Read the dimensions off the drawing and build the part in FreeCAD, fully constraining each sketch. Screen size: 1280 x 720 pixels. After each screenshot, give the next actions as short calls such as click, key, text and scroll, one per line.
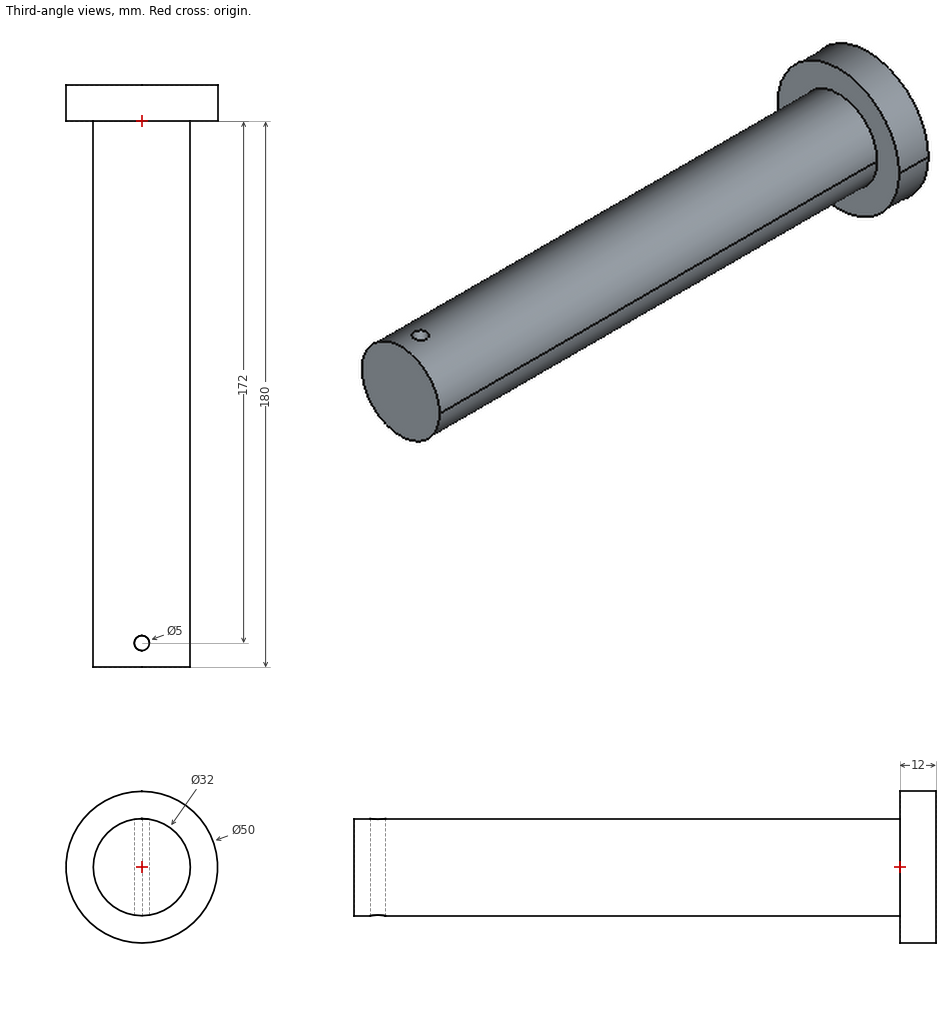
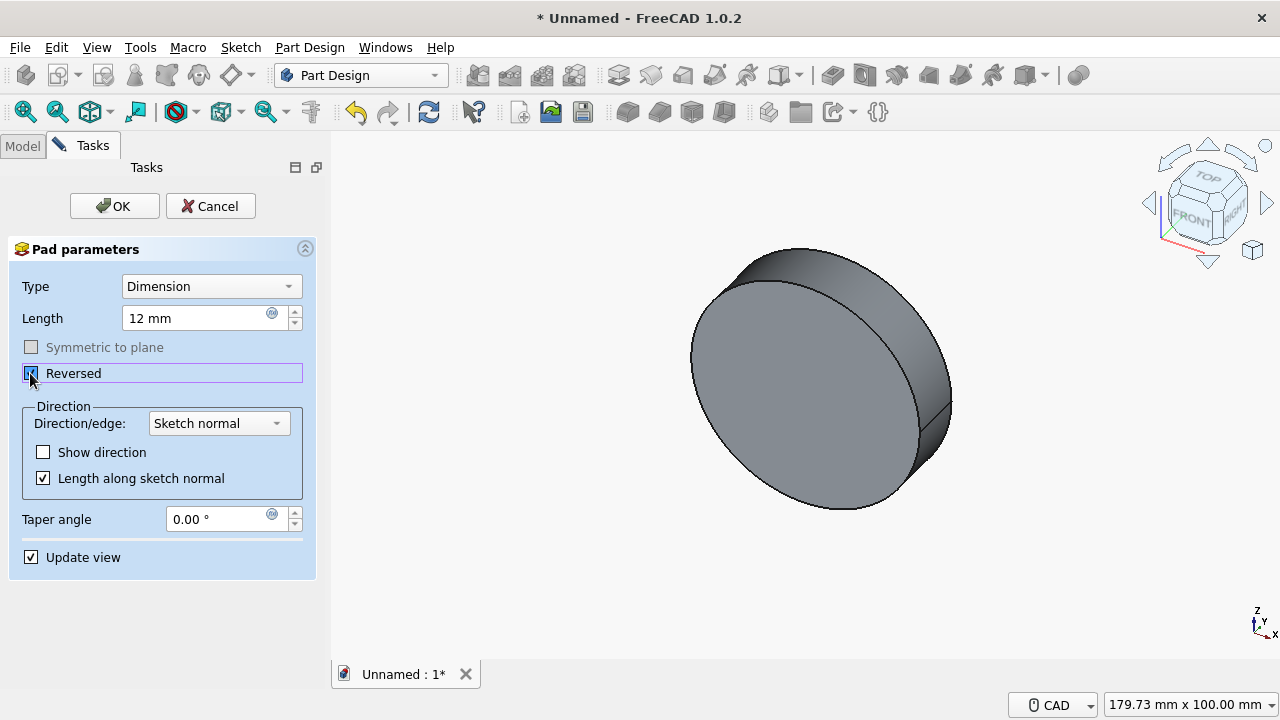
click(115, 206)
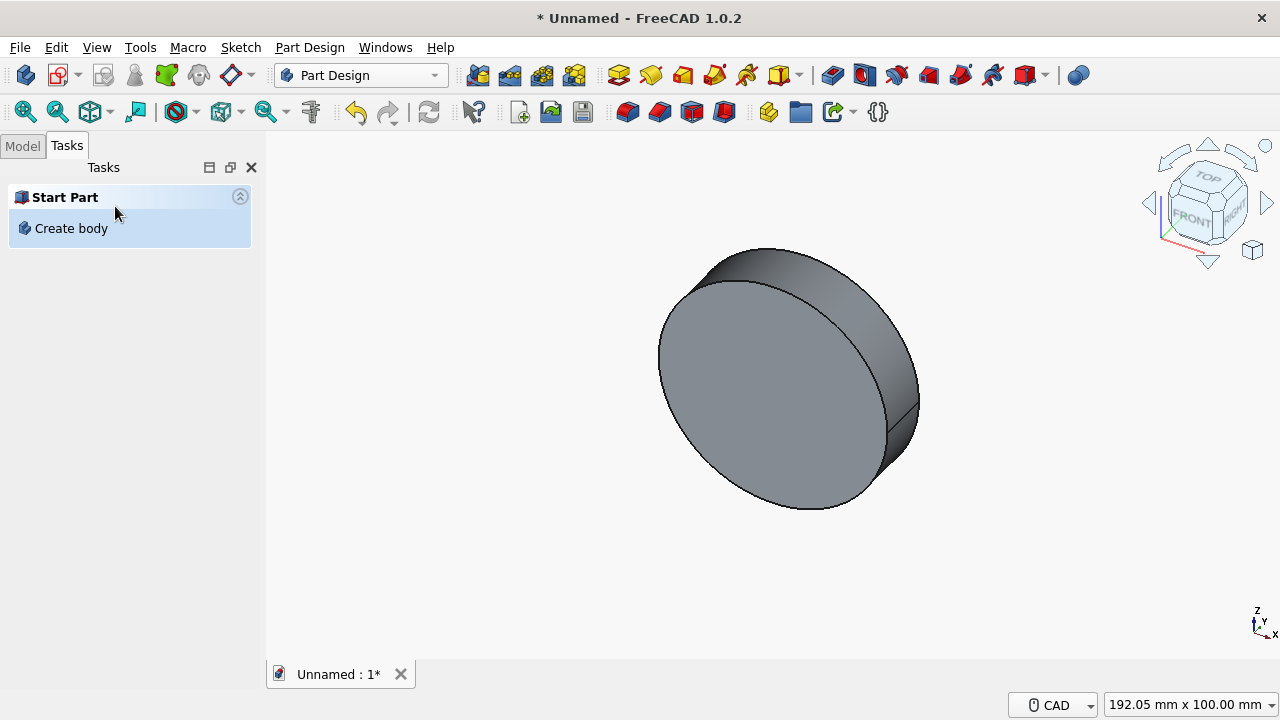
click(58, 76)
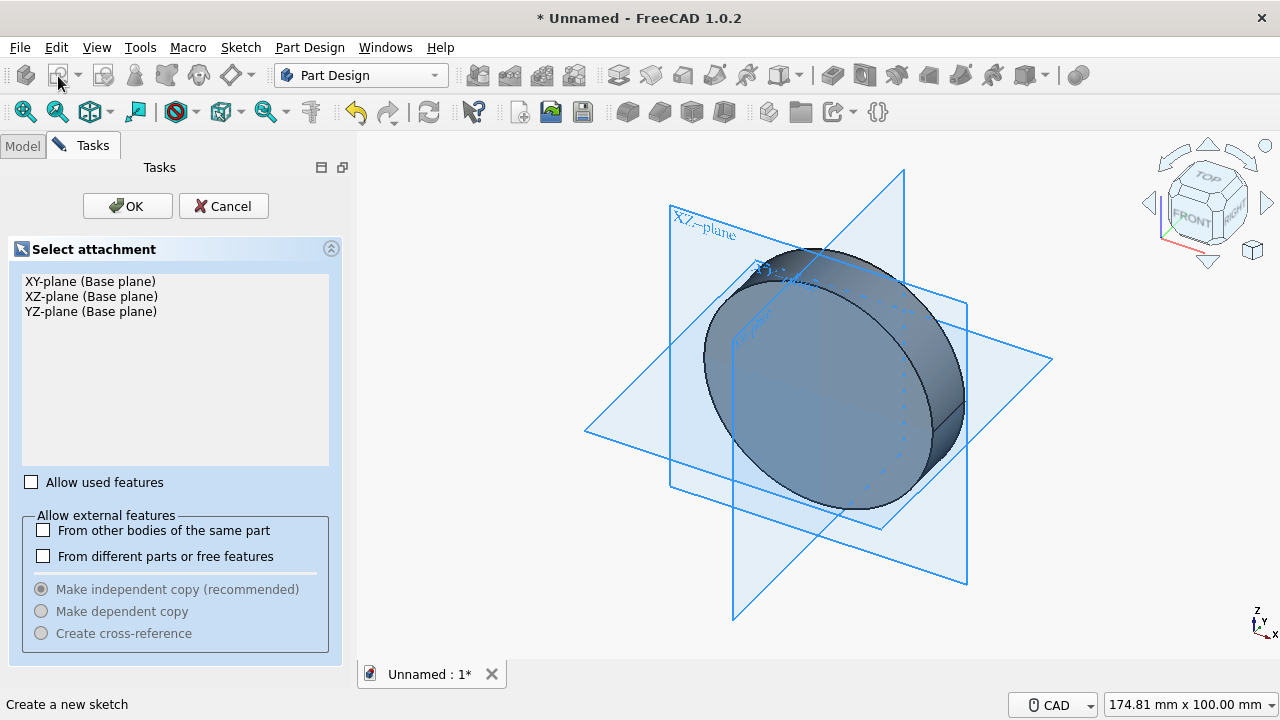
click(82, 296)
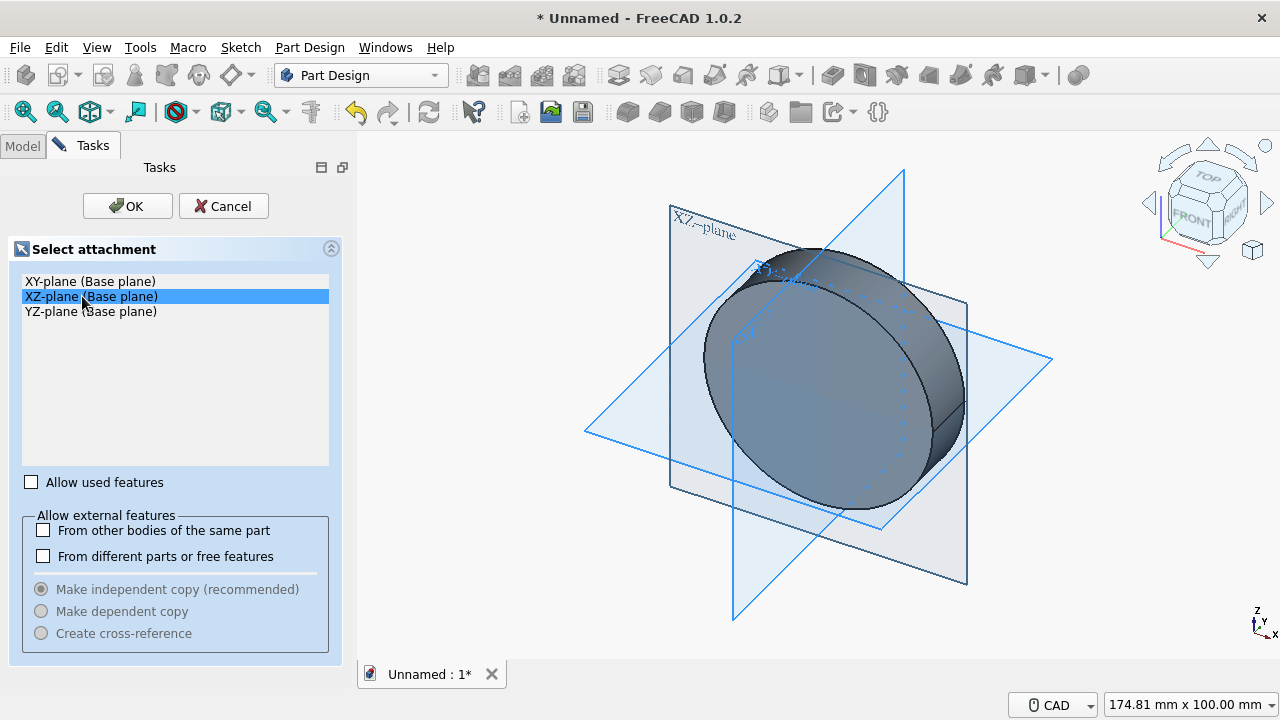
click(128, 206)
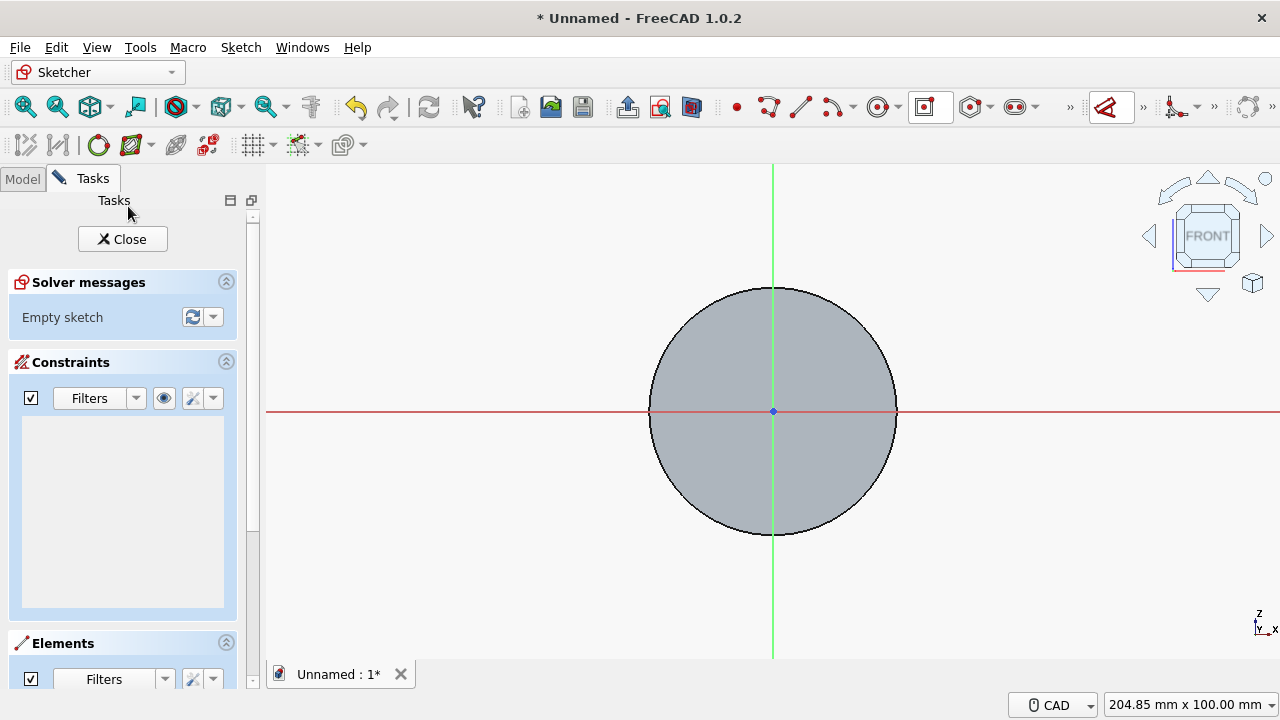
scroll(856, 412, up, 3)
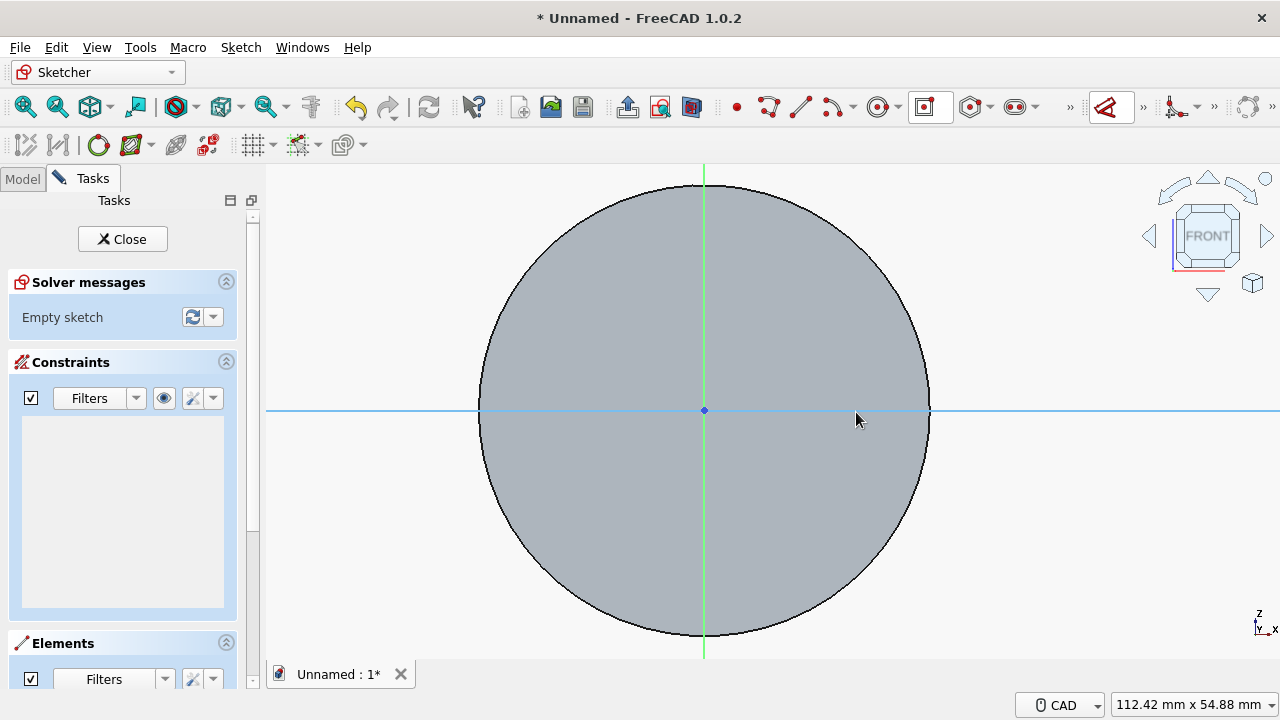
click(878, 108)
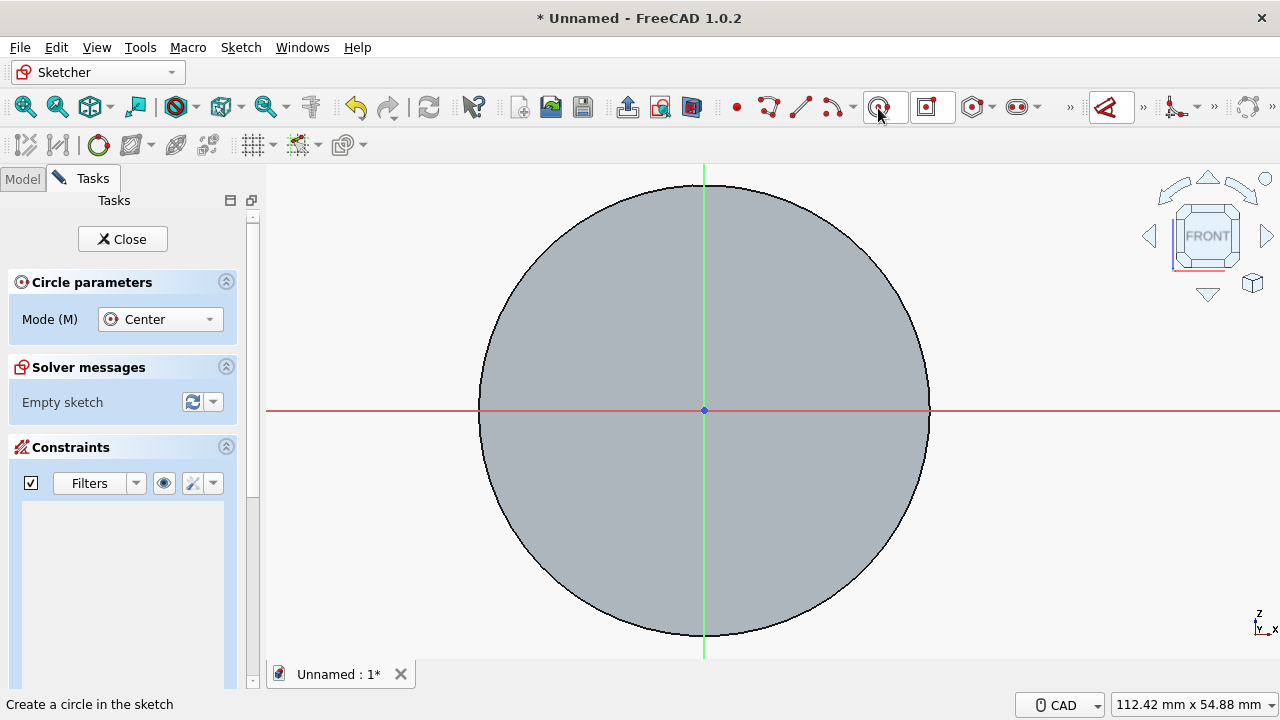
click(704, 411)
move(806, 309)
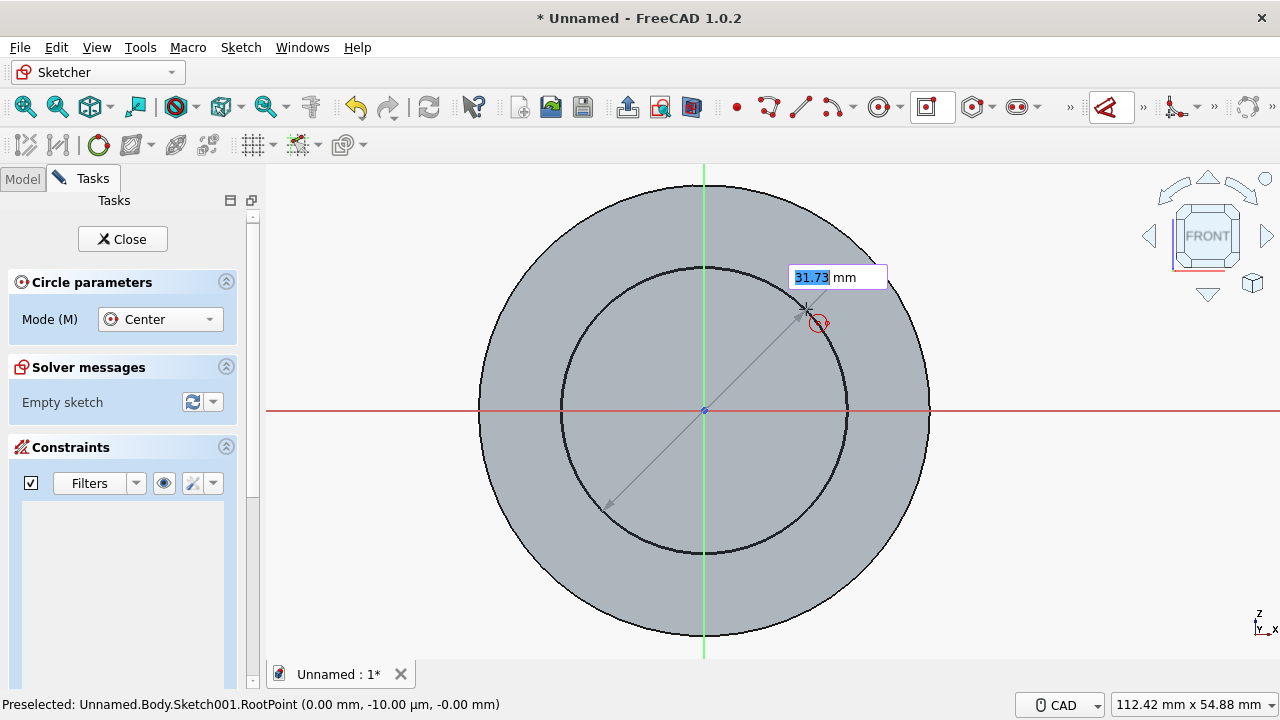
text(32)
key(Return)
key(Escape)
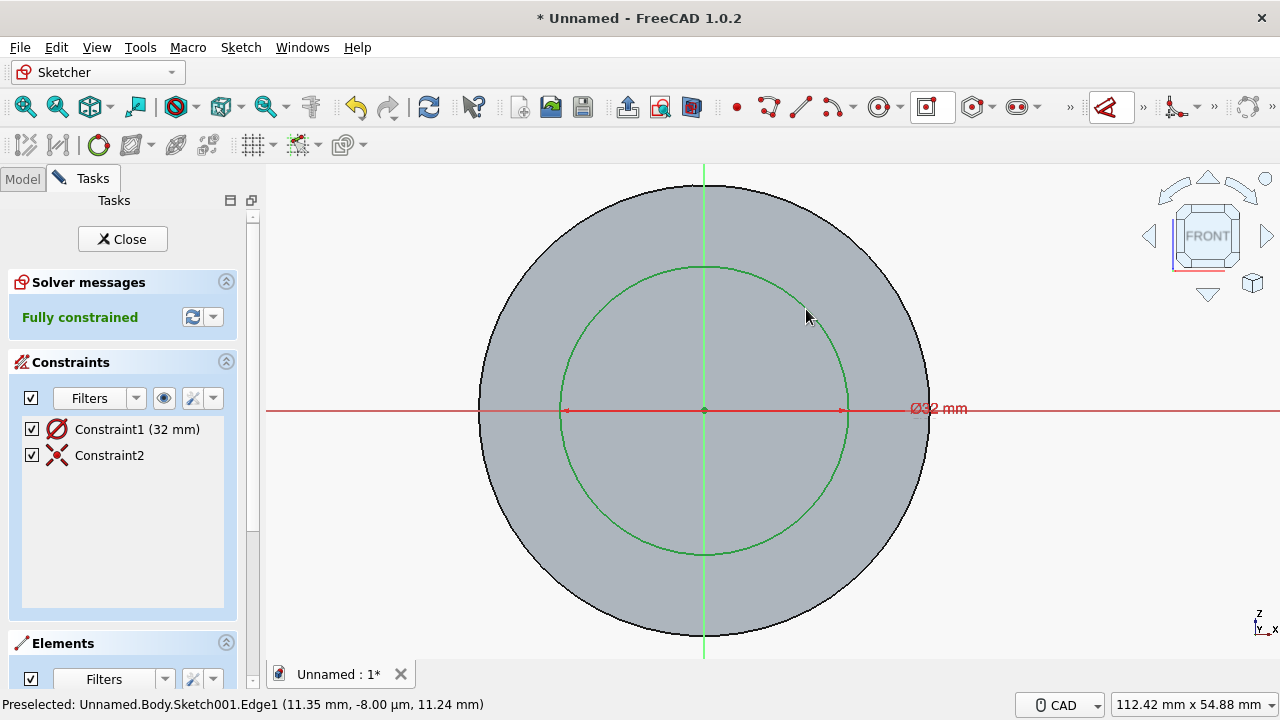
click(123, 239)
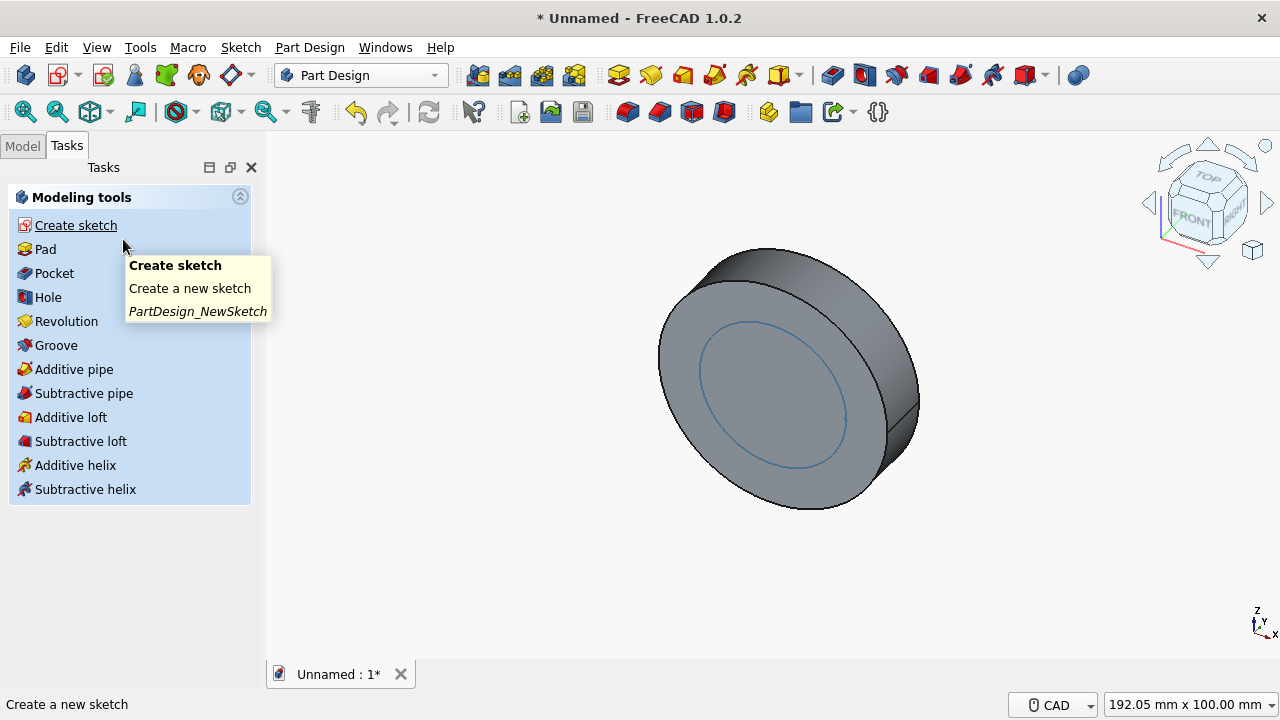
click(620, 76)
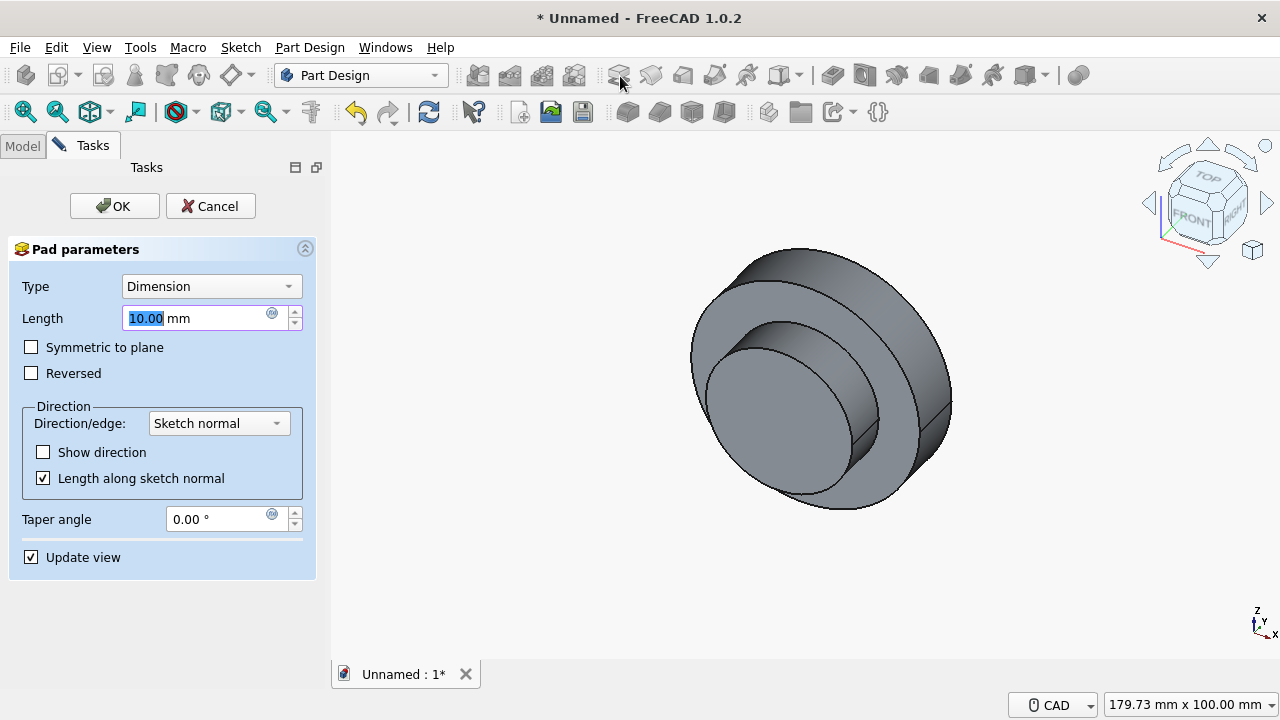
text(180)
key(Tab)